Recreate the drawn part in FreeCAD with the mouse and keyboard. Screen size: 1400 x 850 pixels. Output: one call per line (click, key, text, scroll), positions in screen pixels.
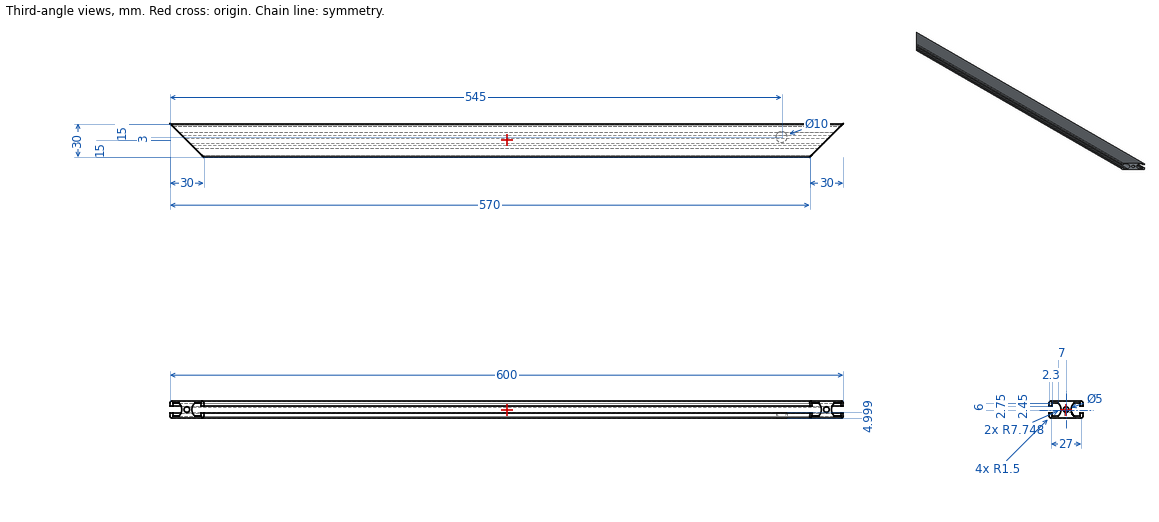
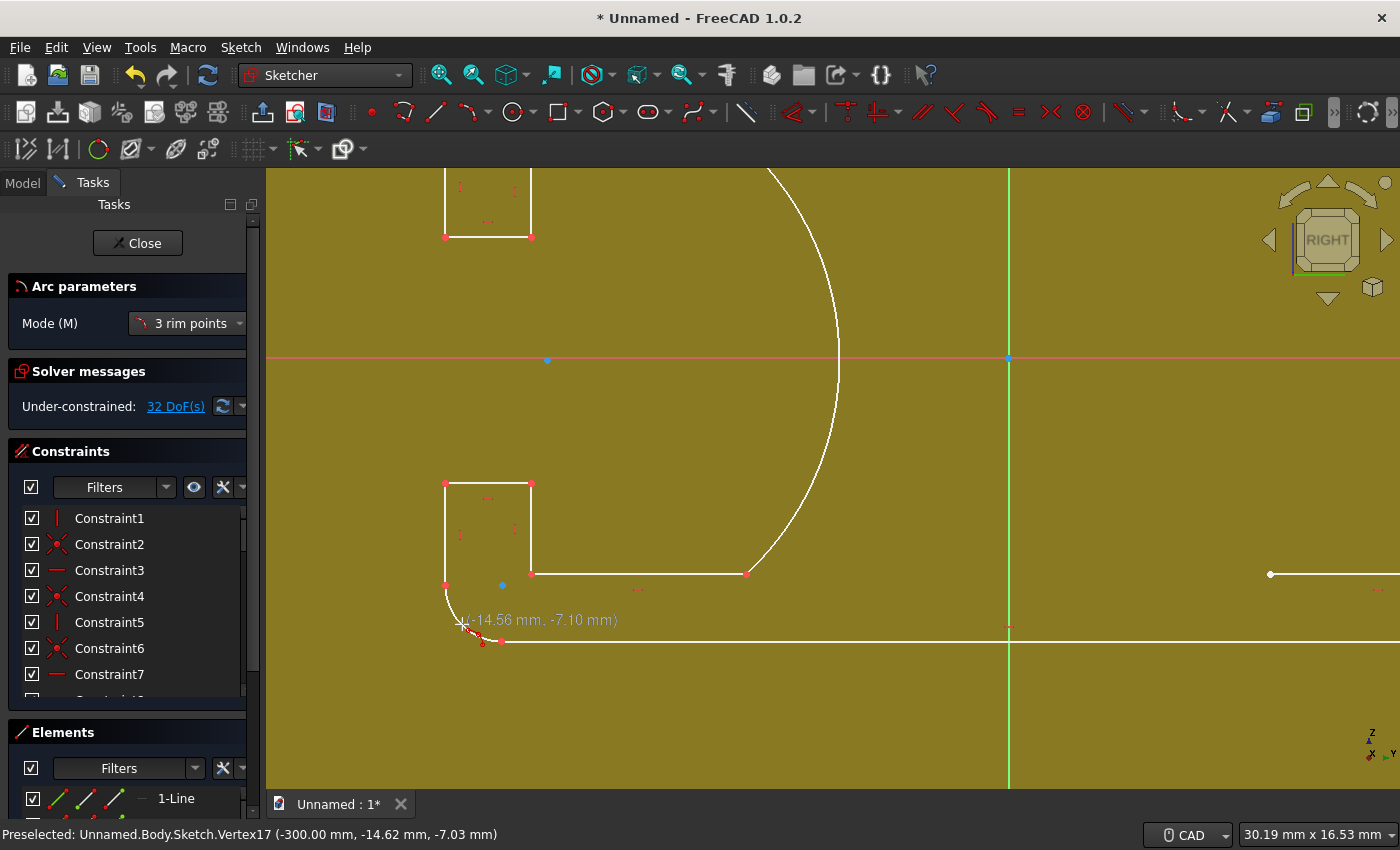
scroll(467, 625, down, 3)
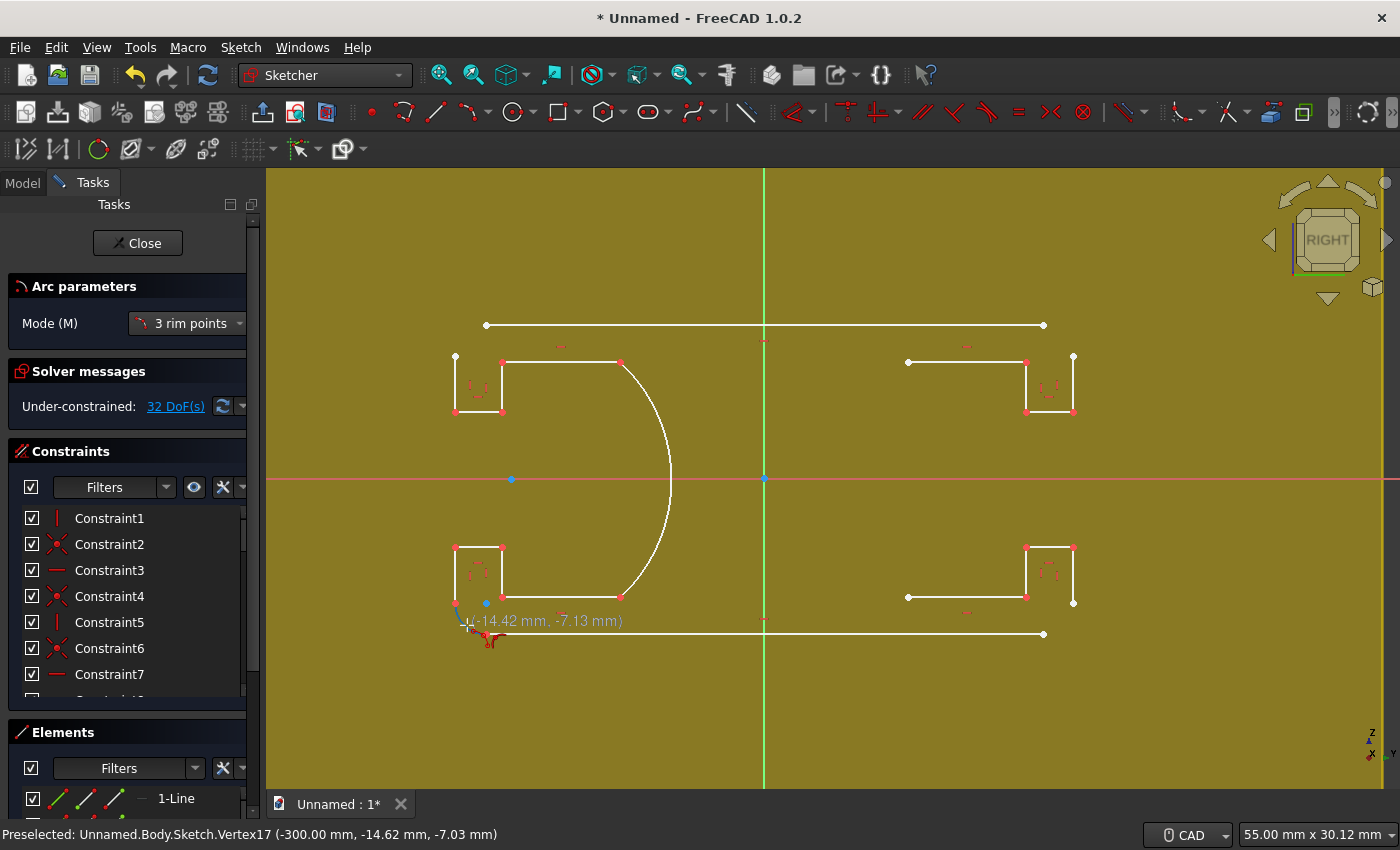
click(1043, 634)
click(1073, 603)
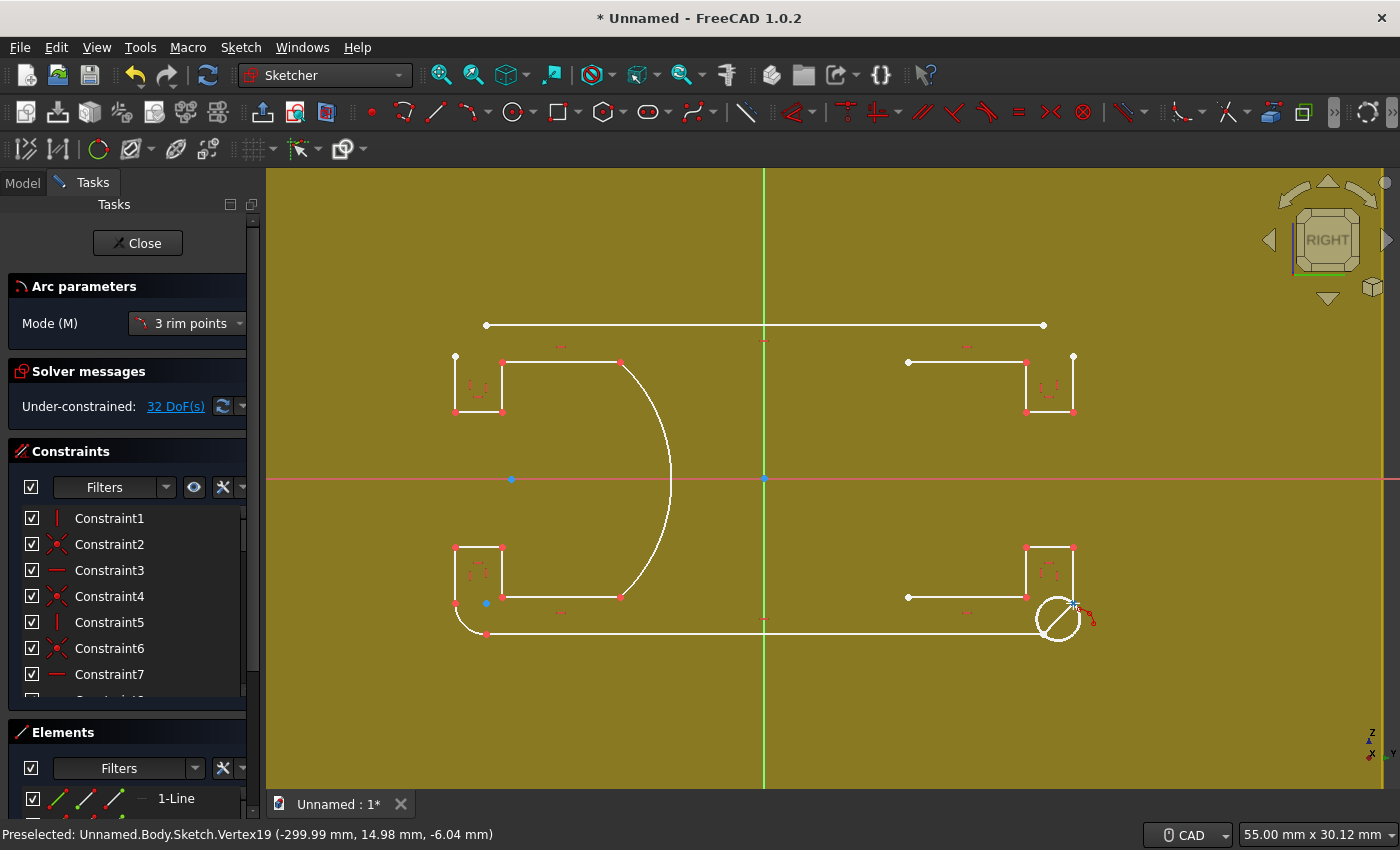
scroll(1065, 625, up, 3)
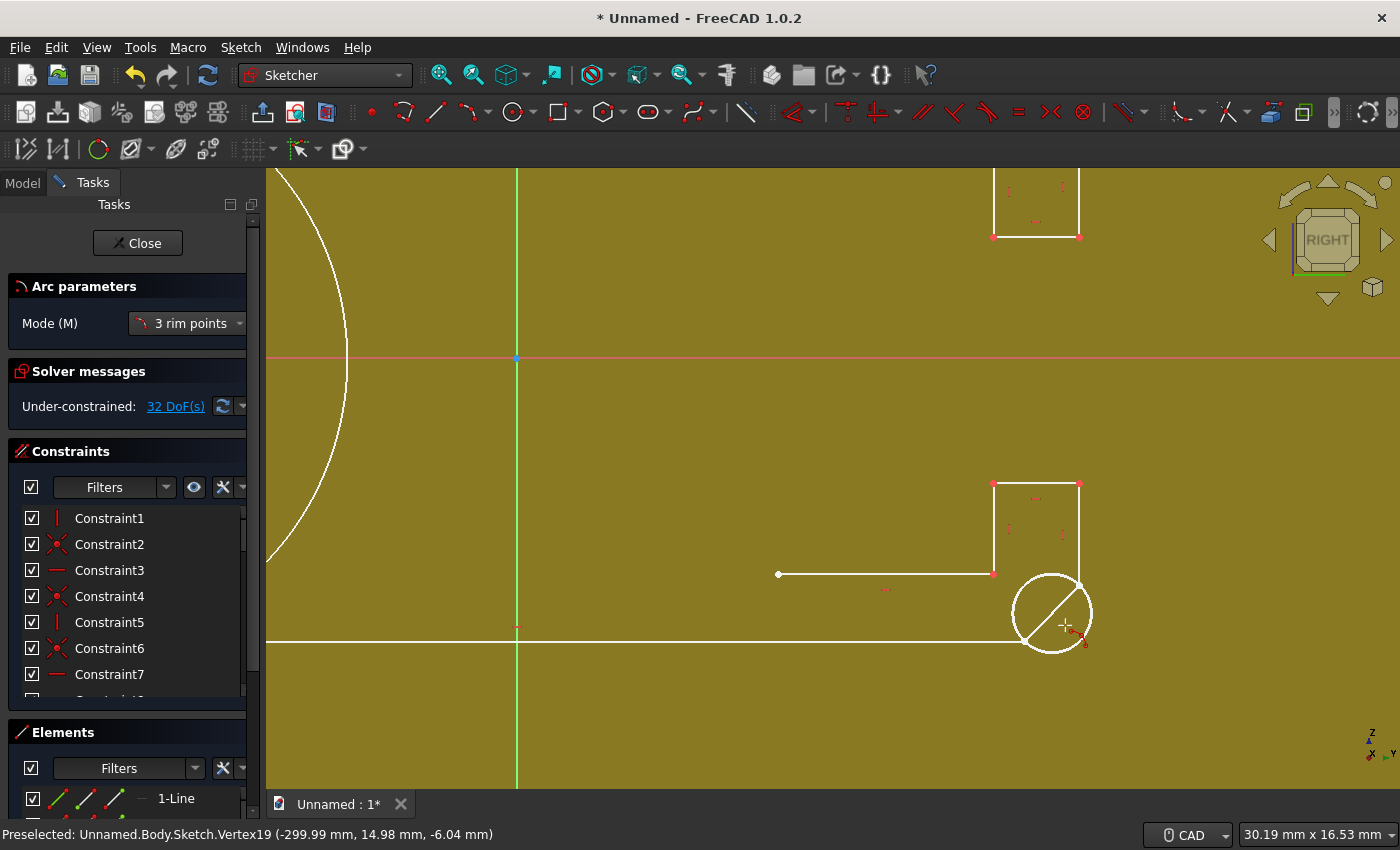
click(1064, 624)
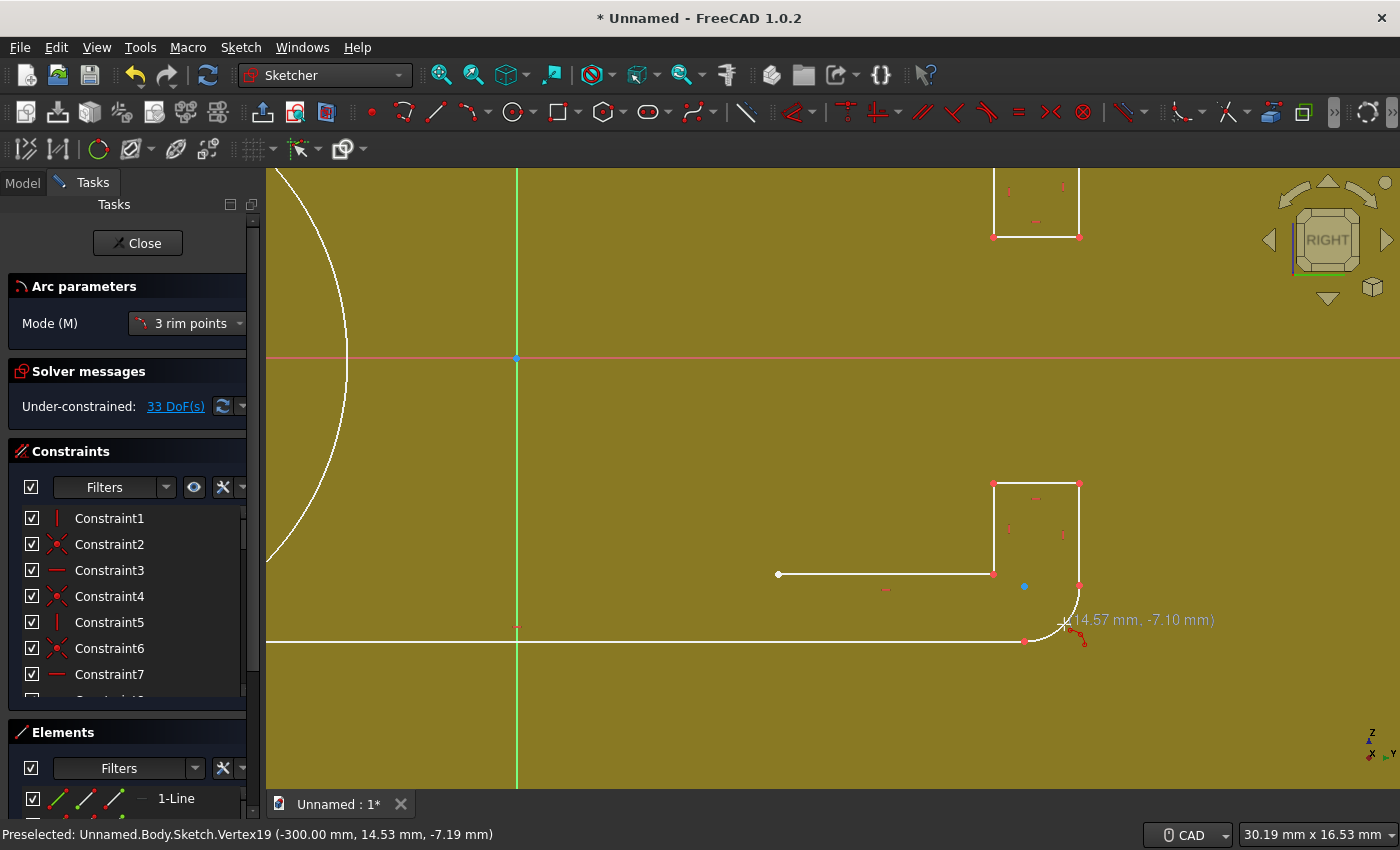
click(779, 574)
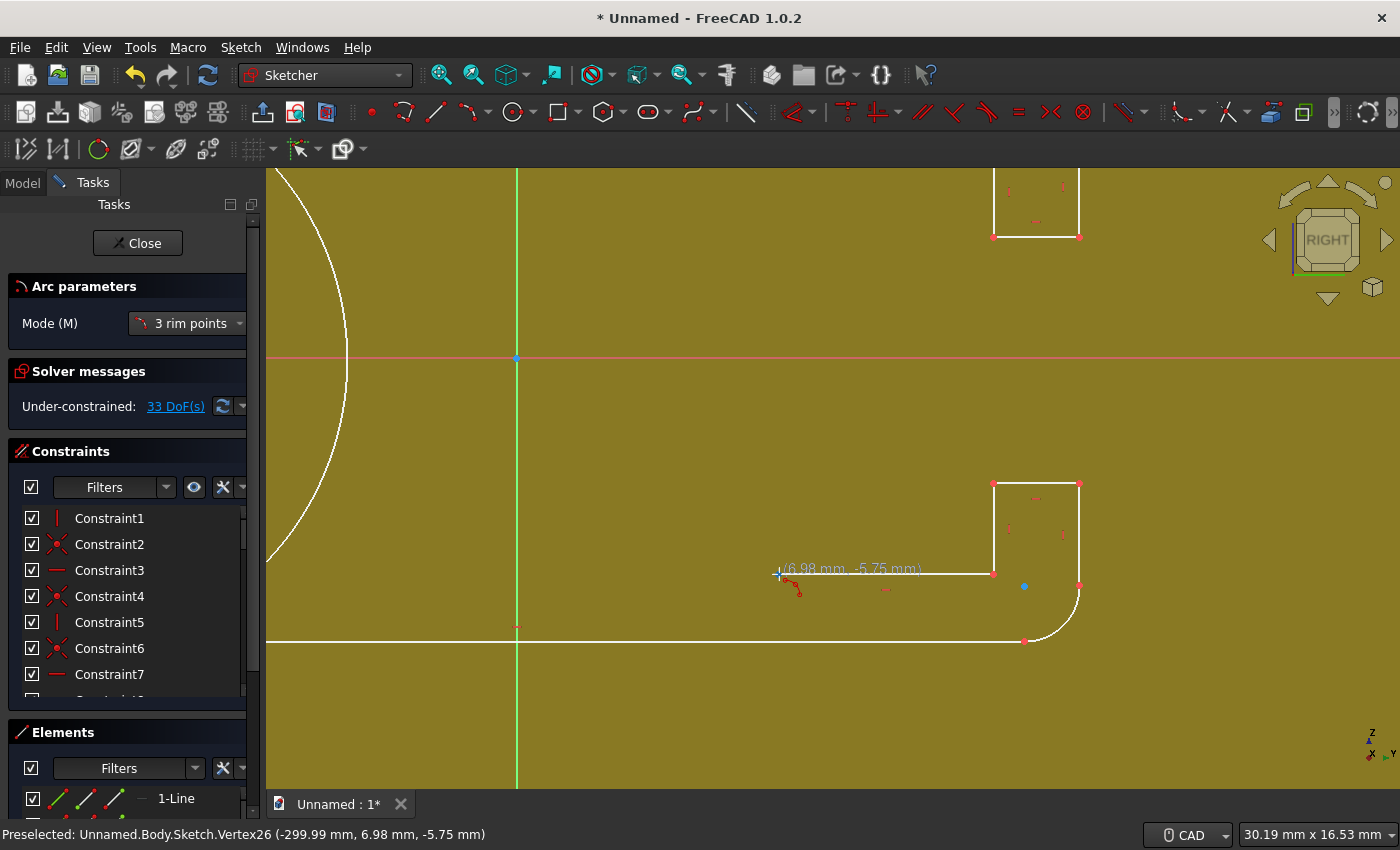
scroll(1066, 625, down, 3)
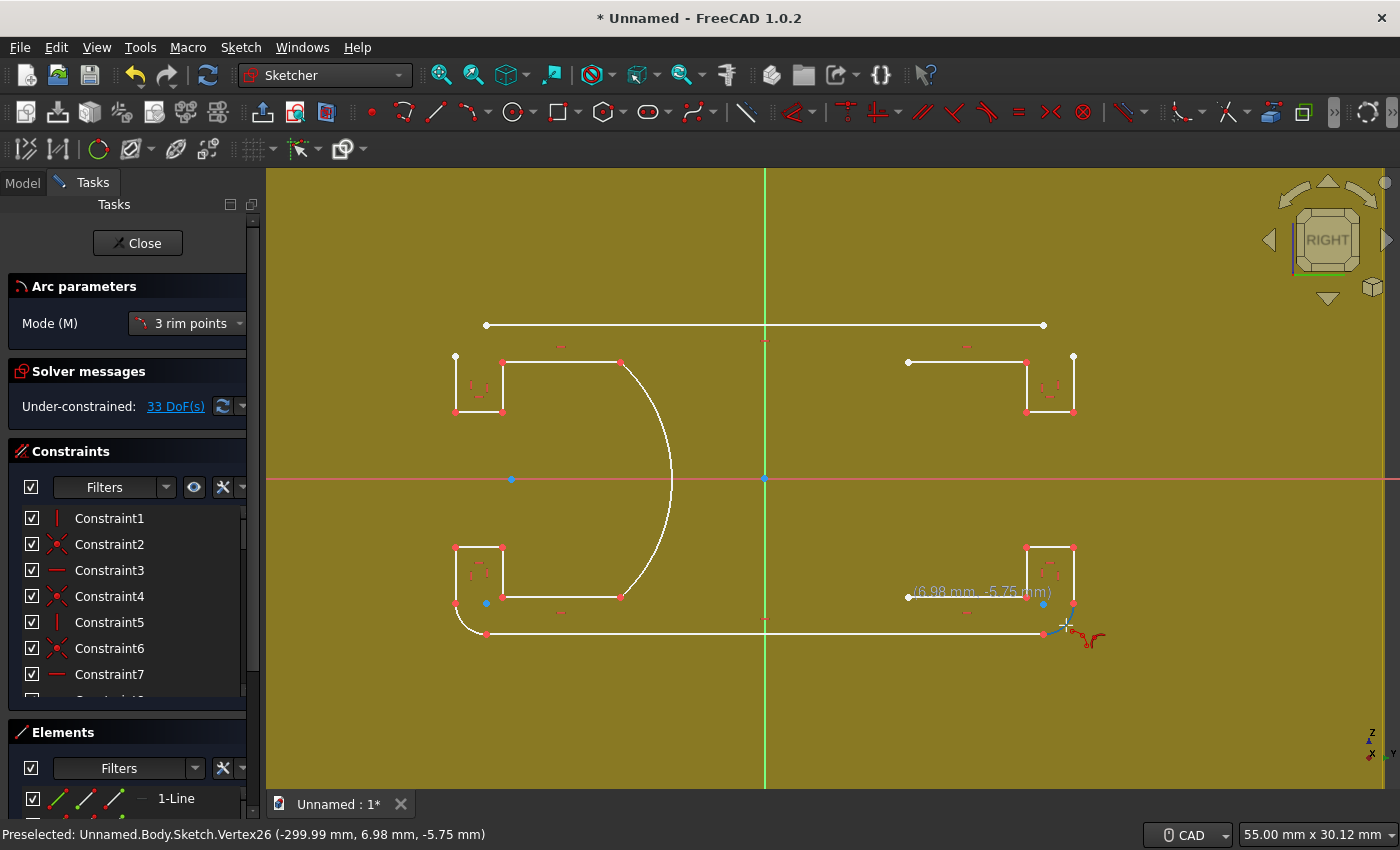
click(909, 362)
click(860, 453)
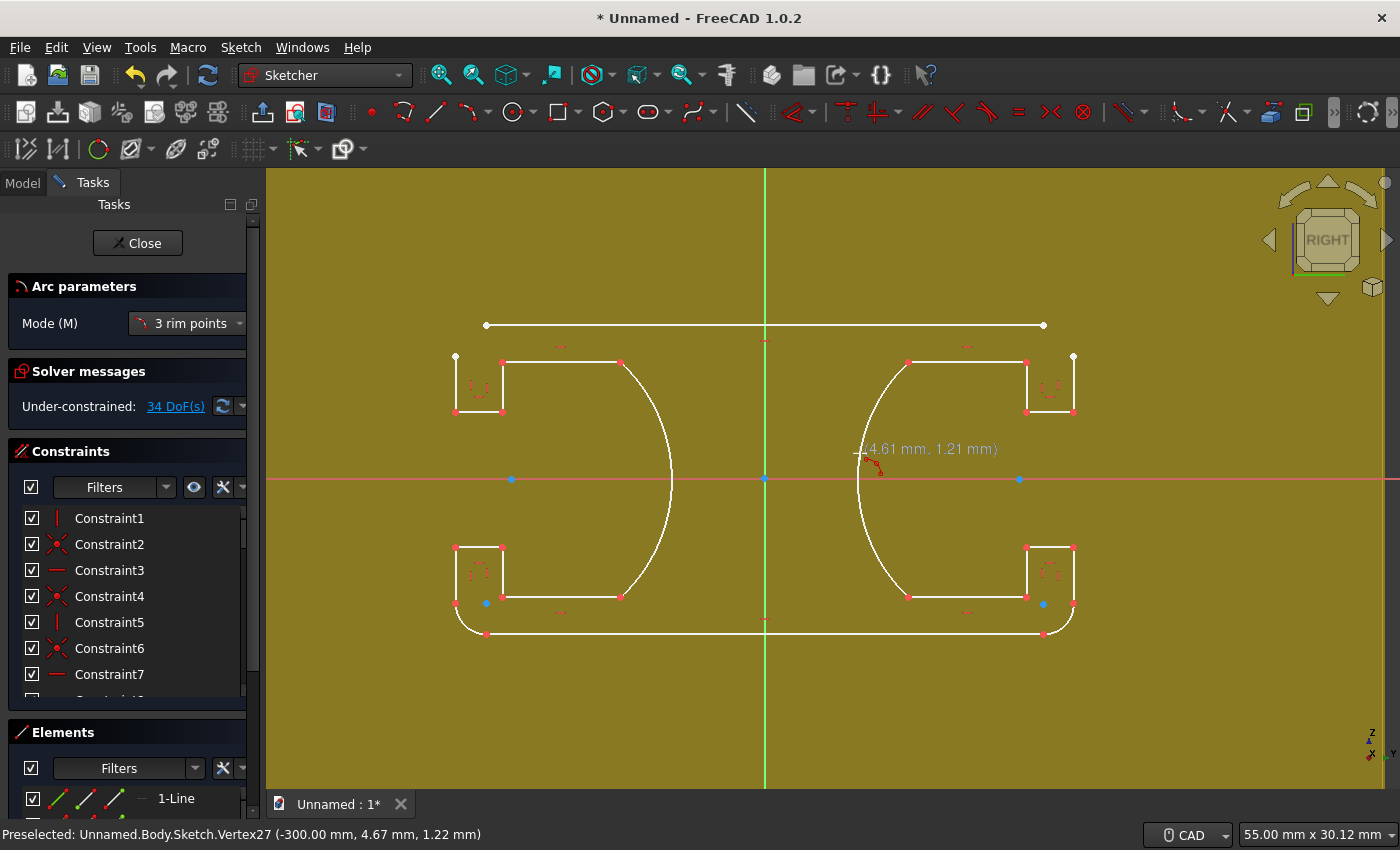
click(1074, 356)
click(1044, 325)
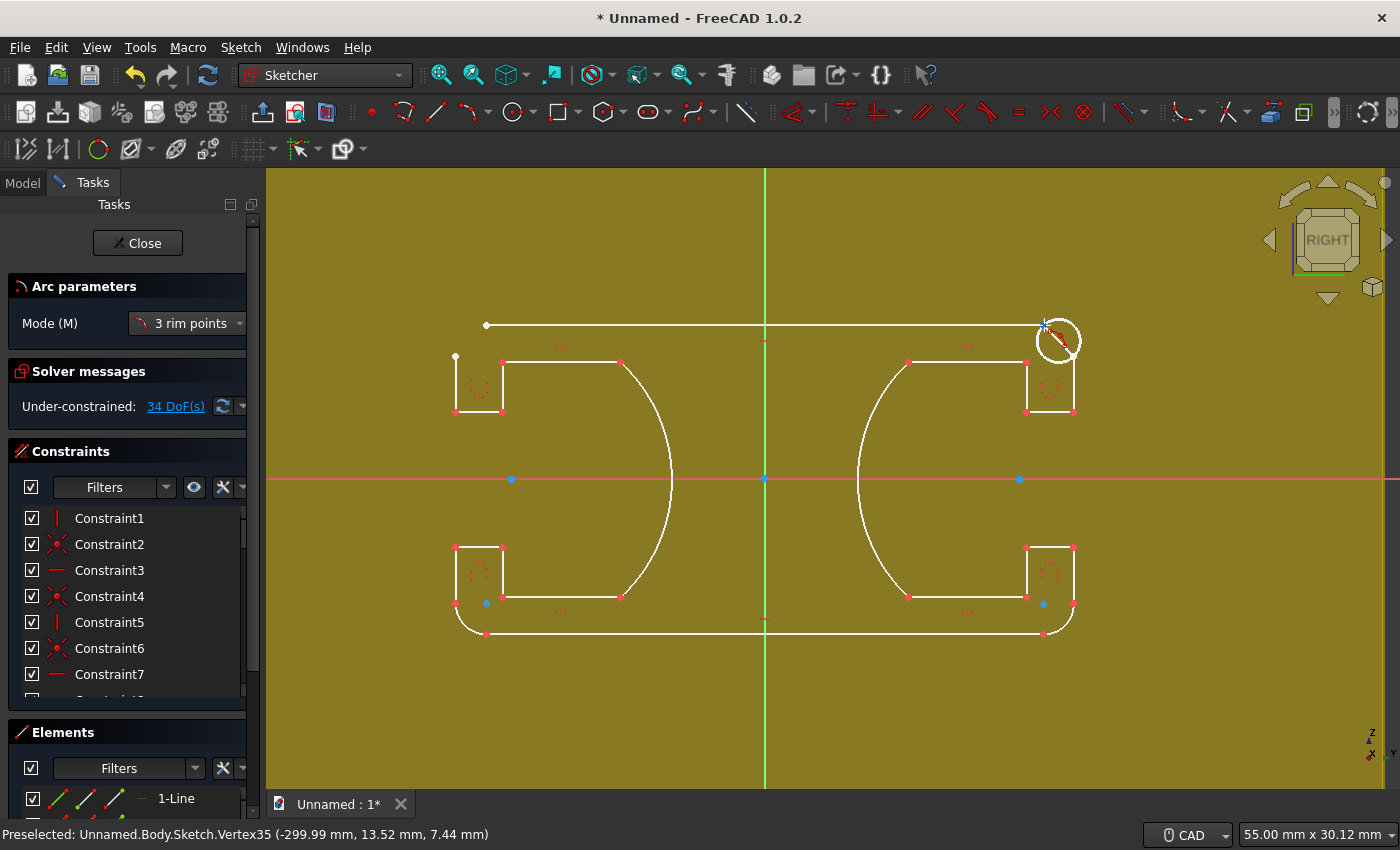
scroll(1065, 333, up, 3)